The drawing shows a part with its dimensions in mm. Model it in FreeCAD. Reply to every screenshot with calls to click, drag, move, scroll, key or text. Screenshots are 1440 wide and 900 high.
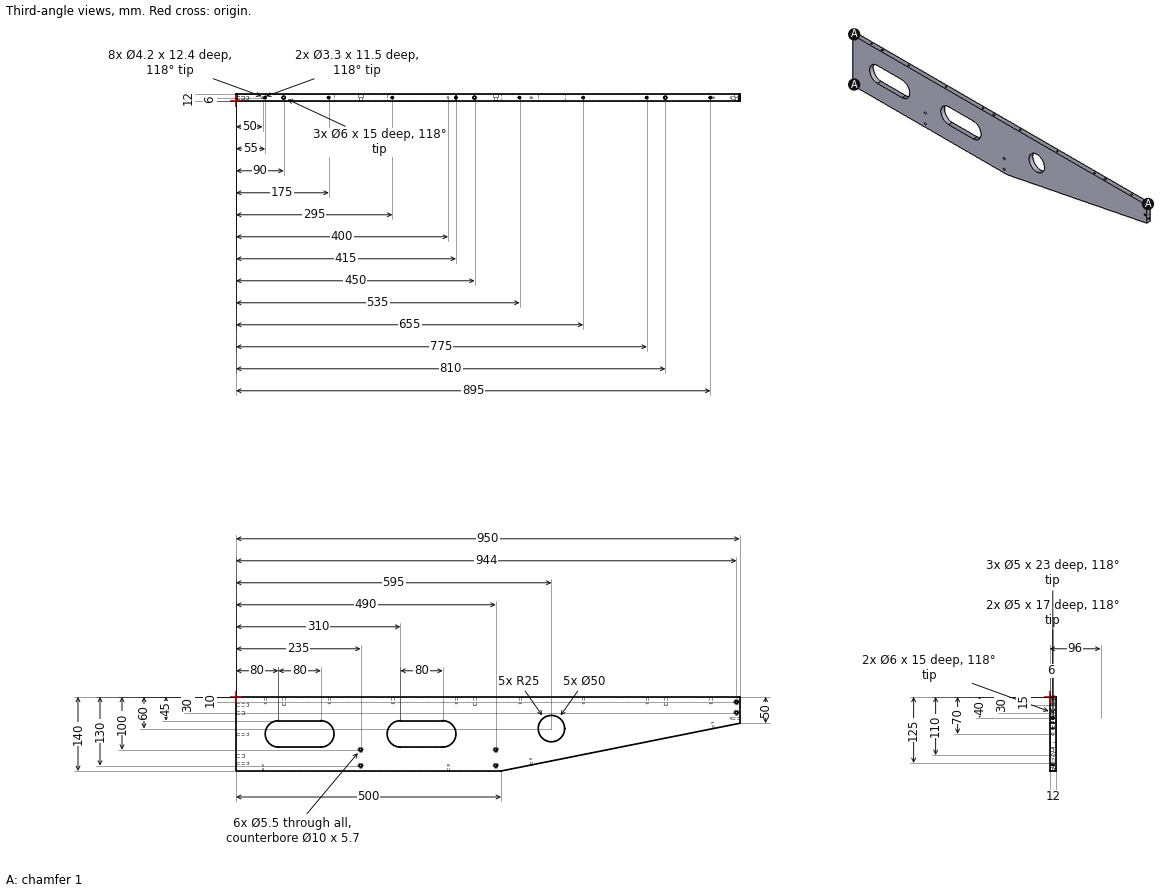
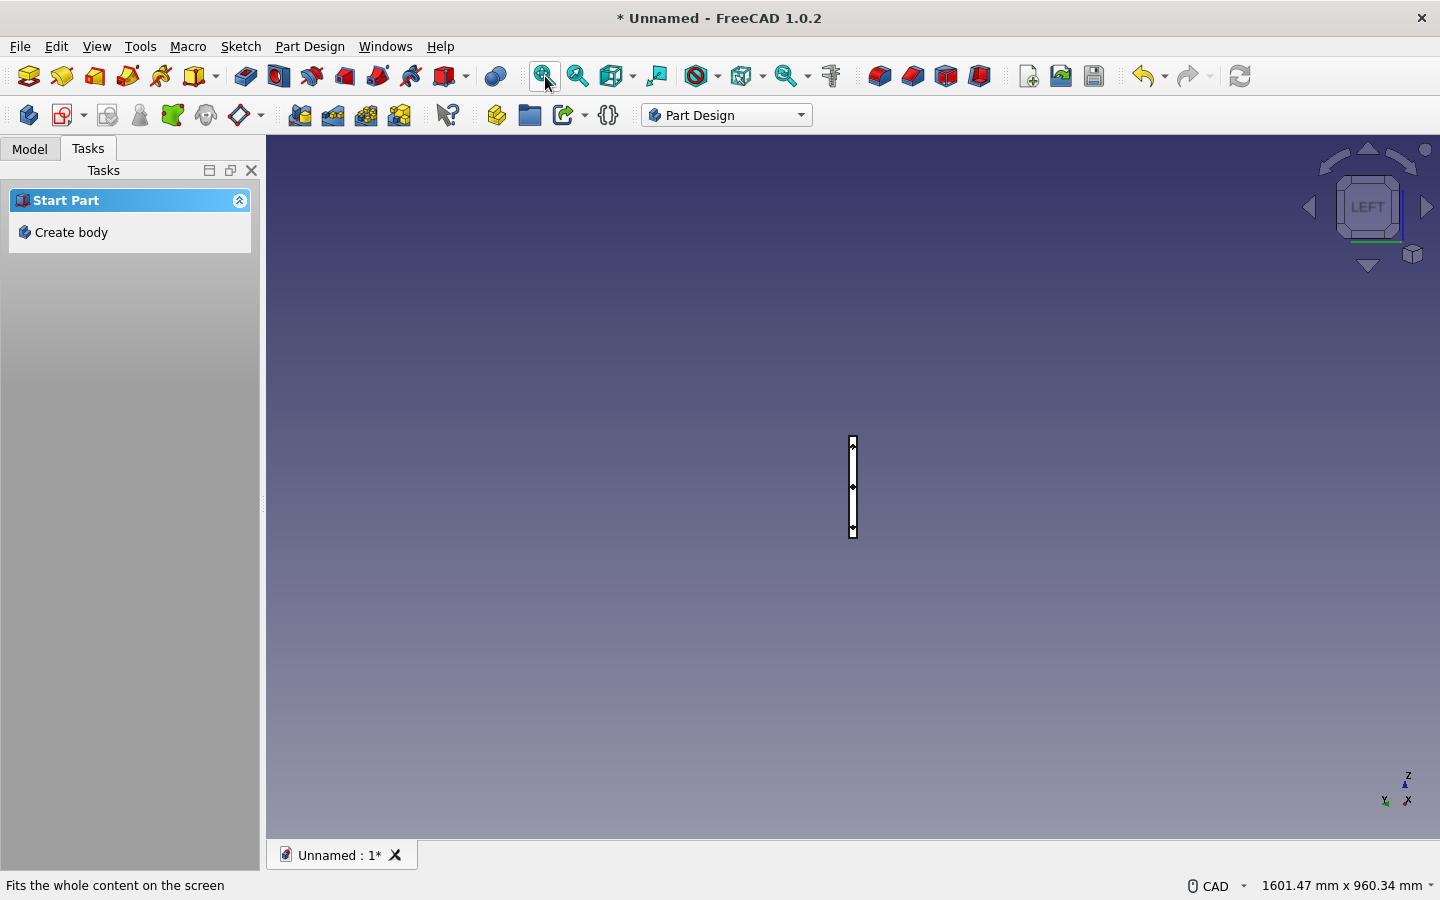
scroll(853, 457, up, 6)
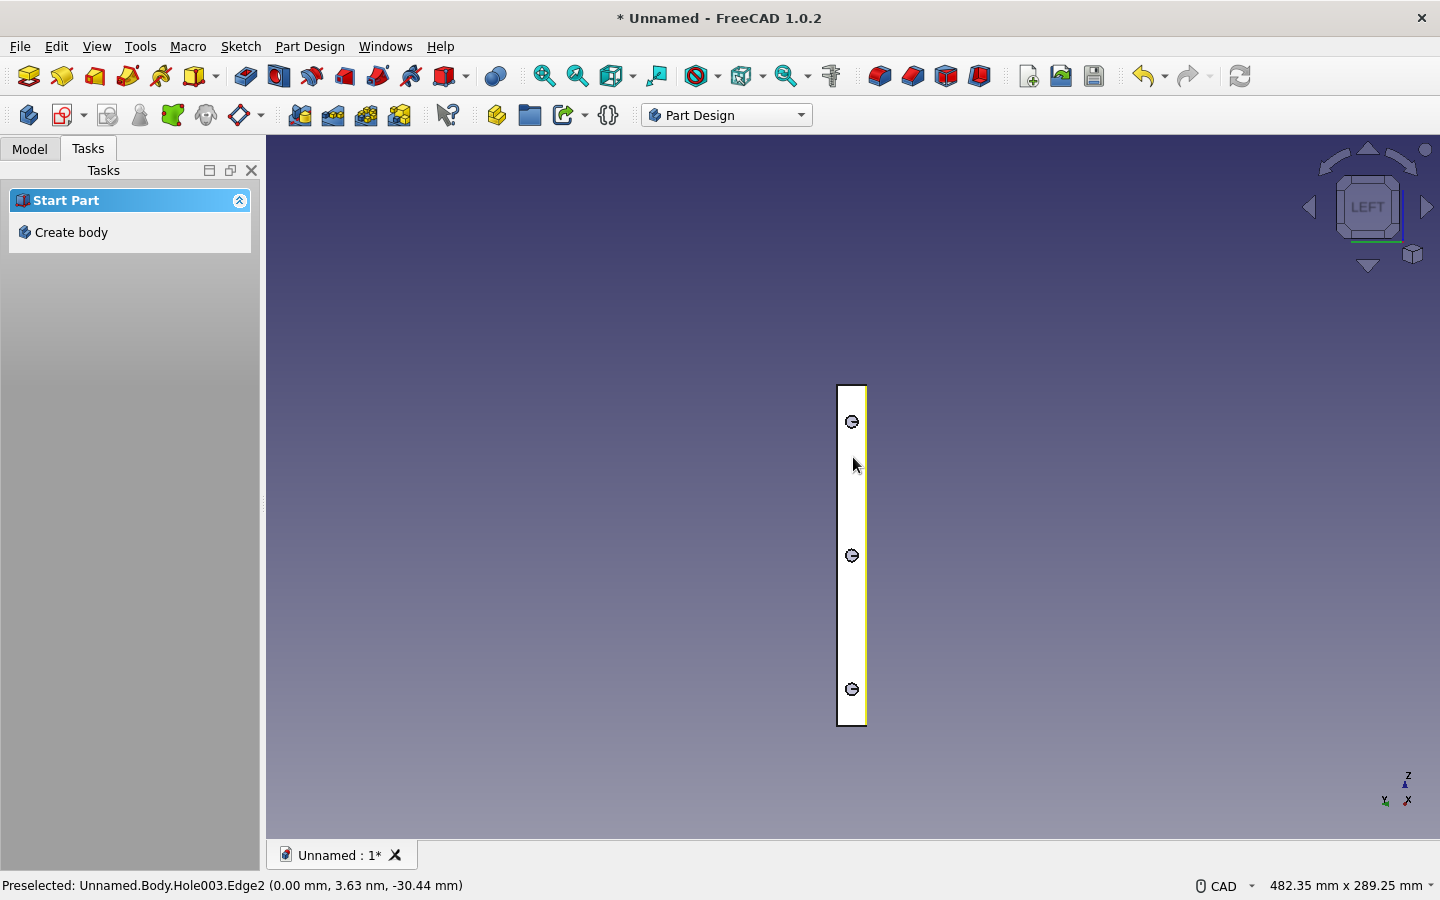
click(852, 457)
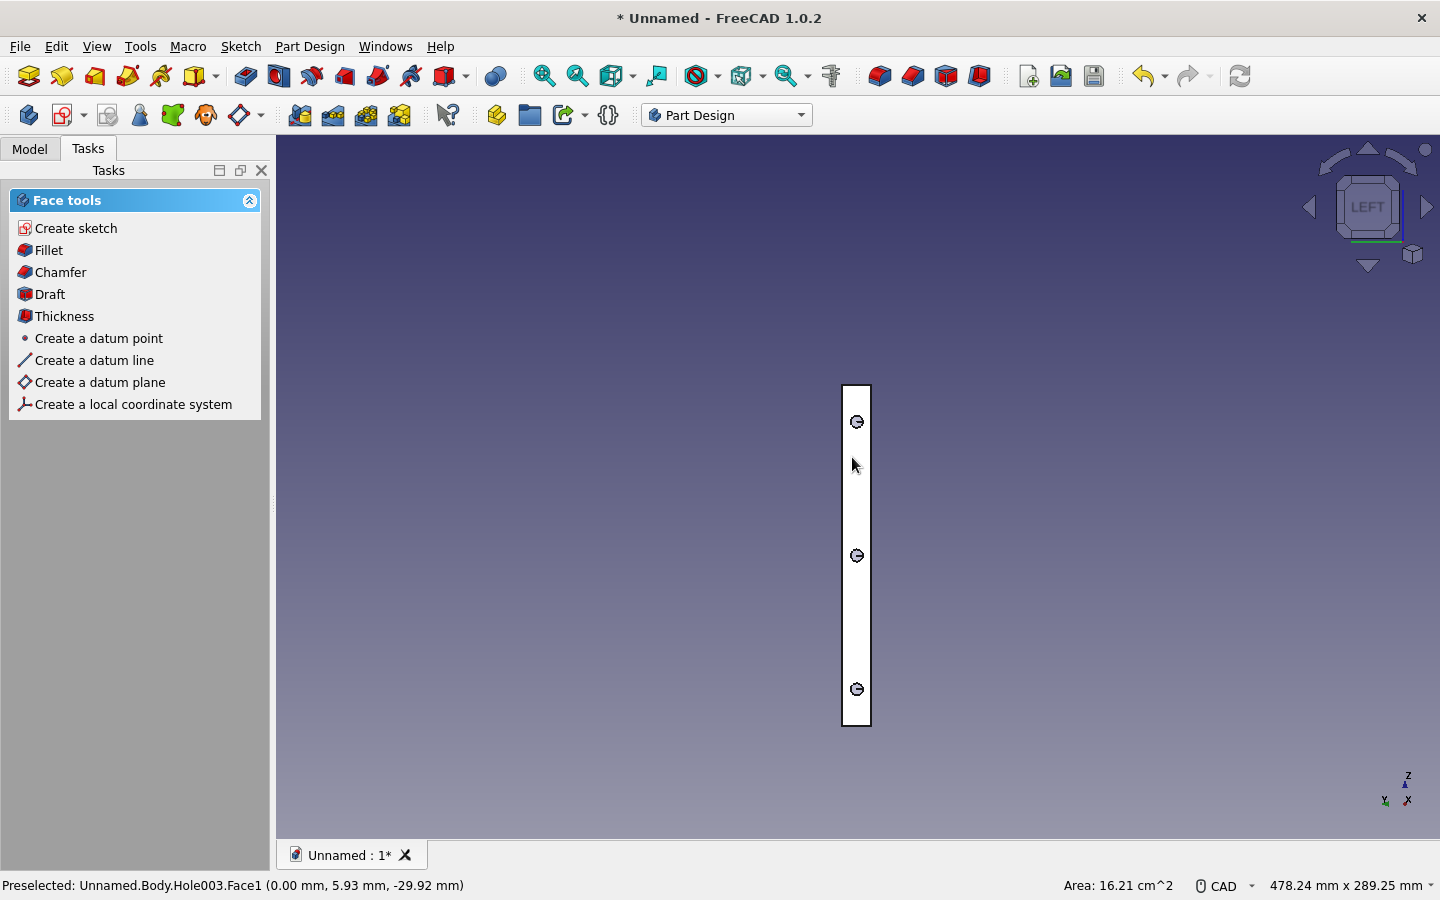
click(62, 116)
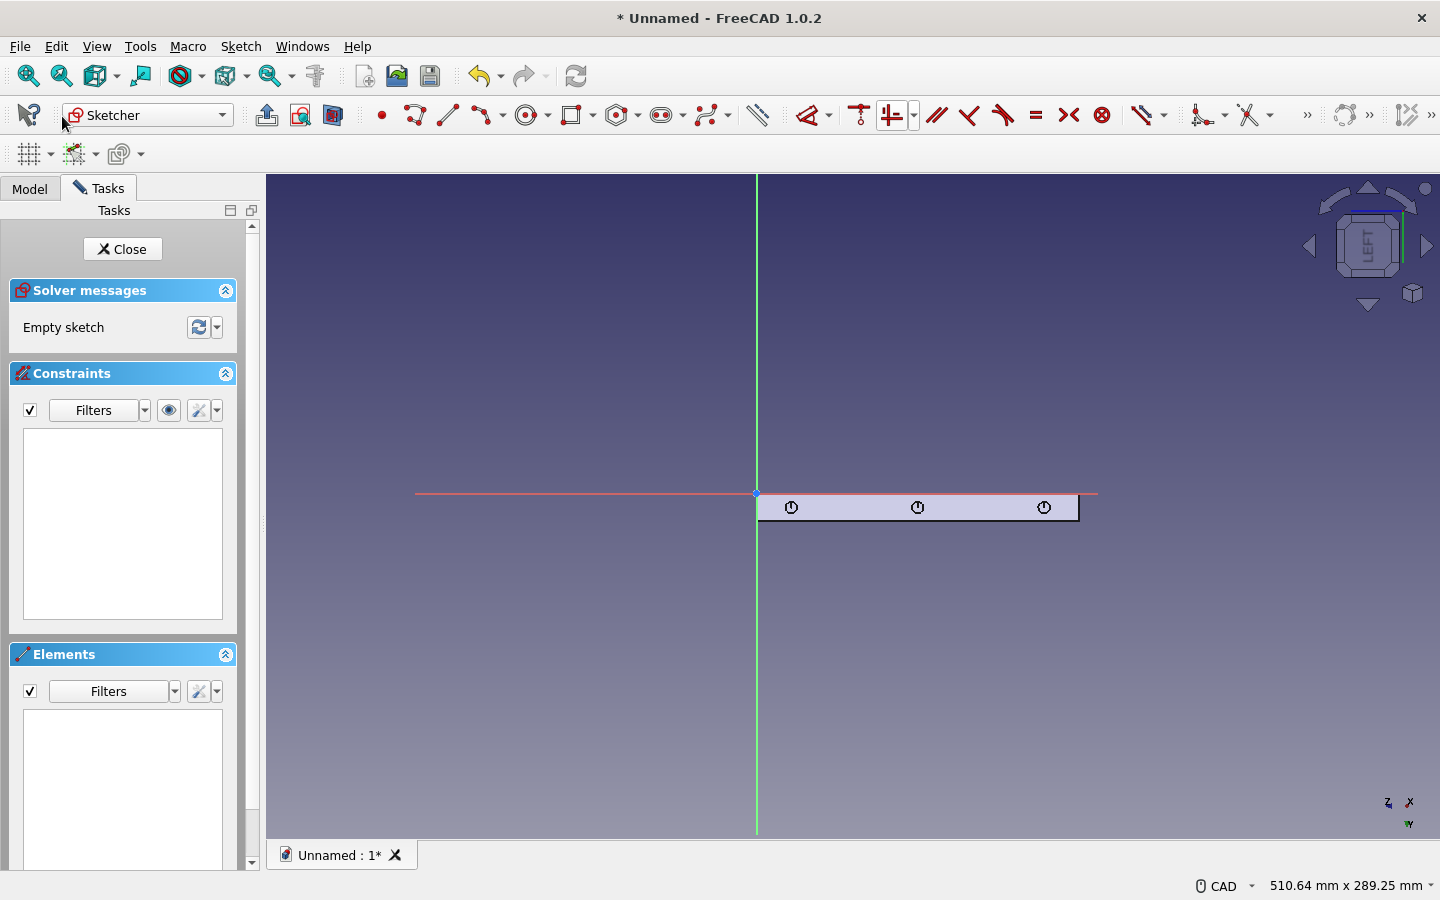
scroll(946, 503, up, 5)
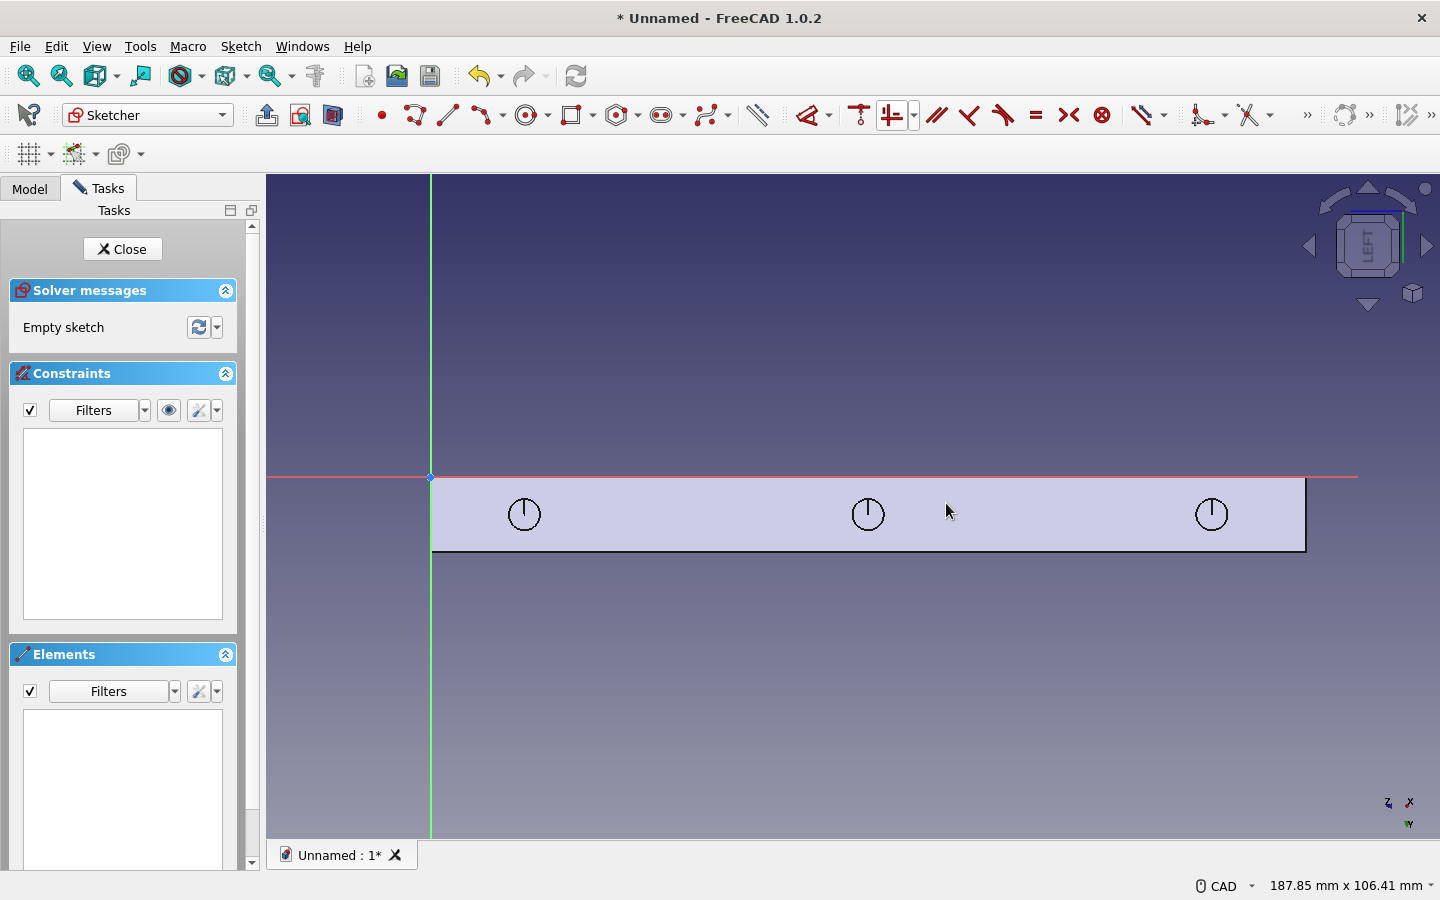
click(526, 116)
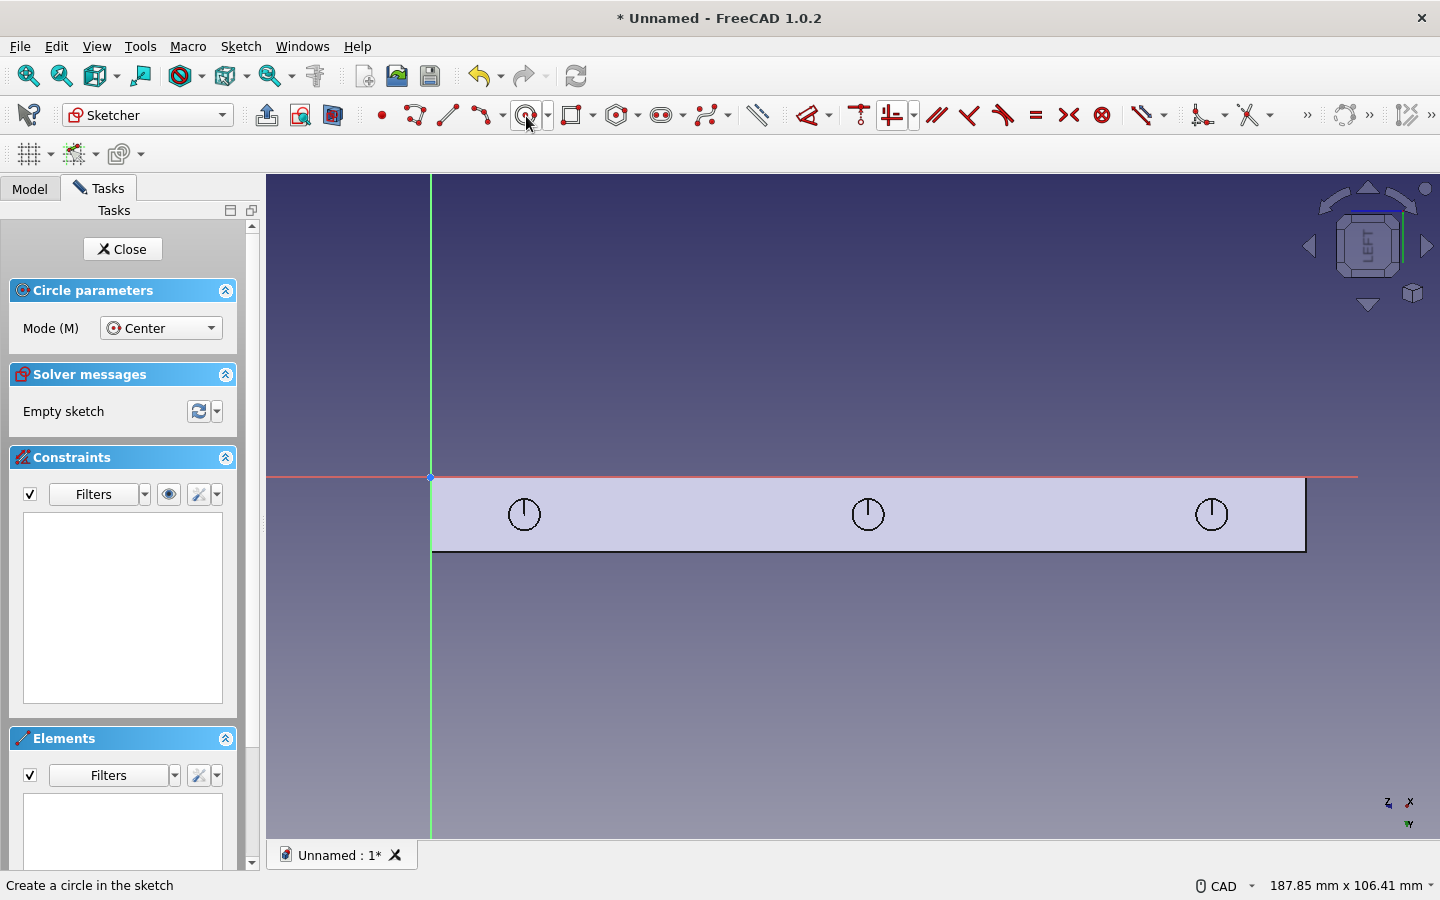
click(618, 515)
move(631, 501)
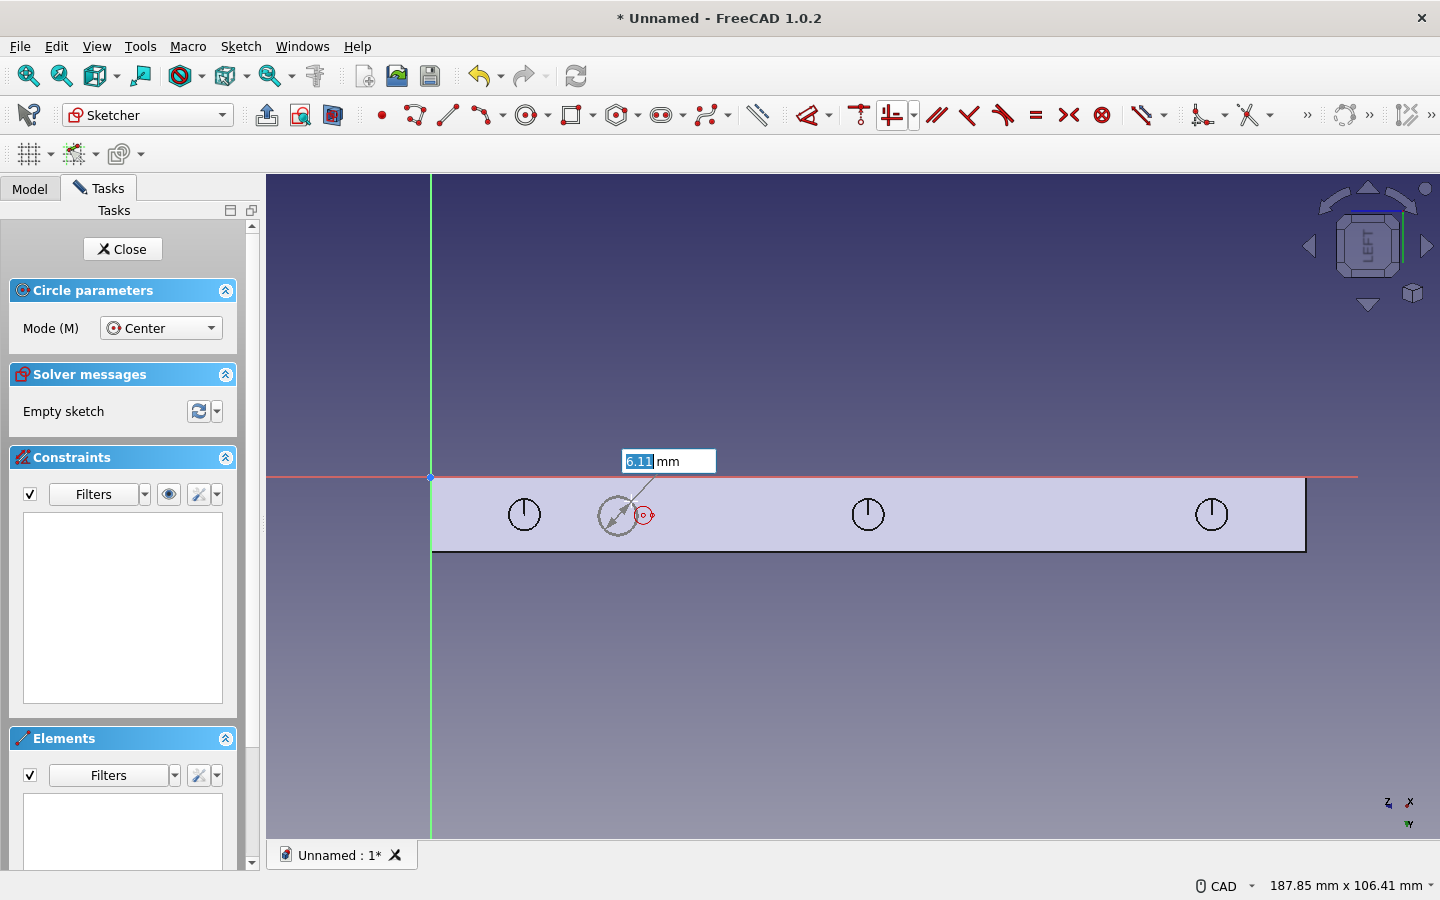
text(6)
key(Return)